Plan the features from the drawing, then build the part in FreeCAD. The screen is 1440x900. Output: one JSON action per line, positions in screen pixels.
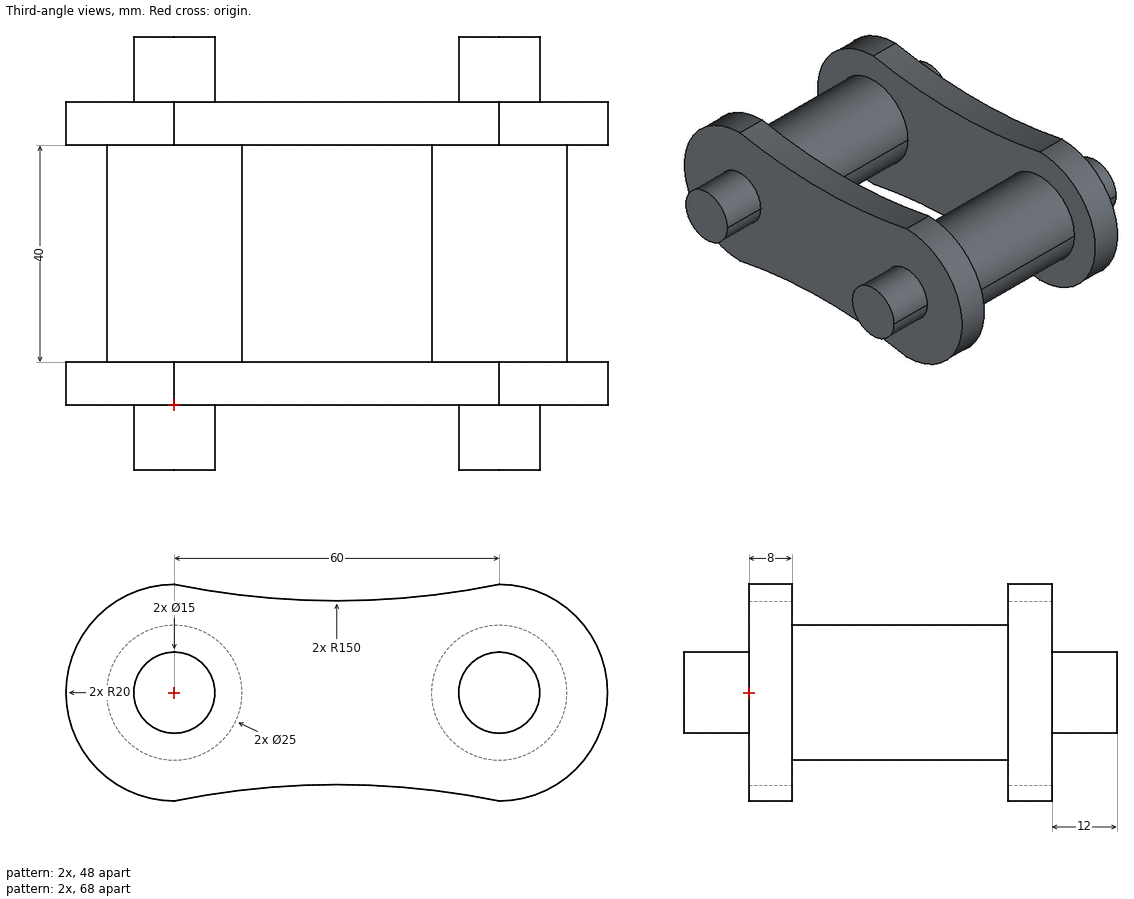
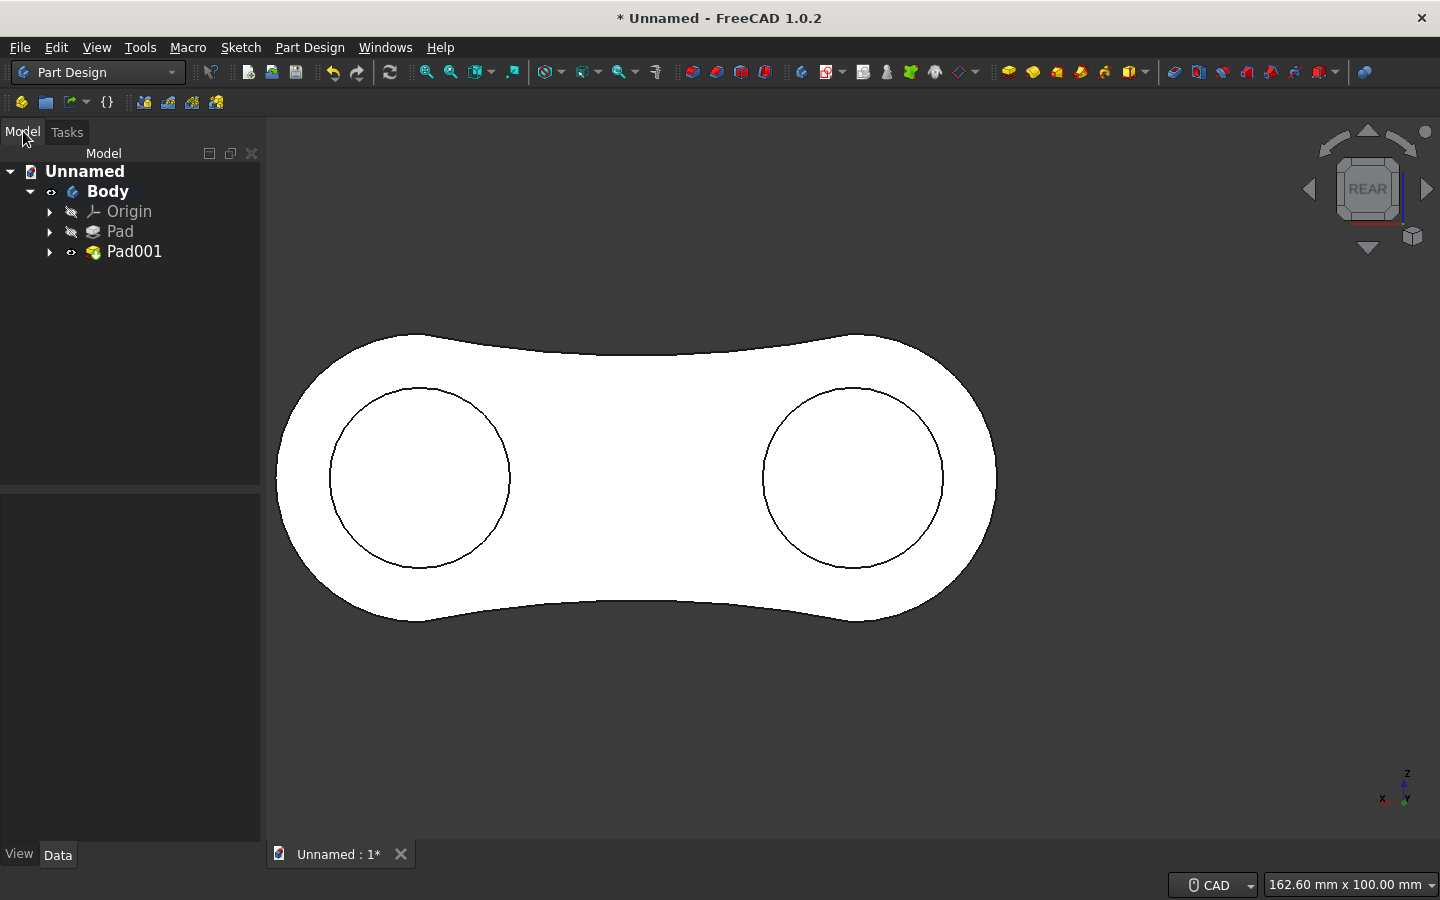
{"action": "left_click", "coordinate": [116, 232]}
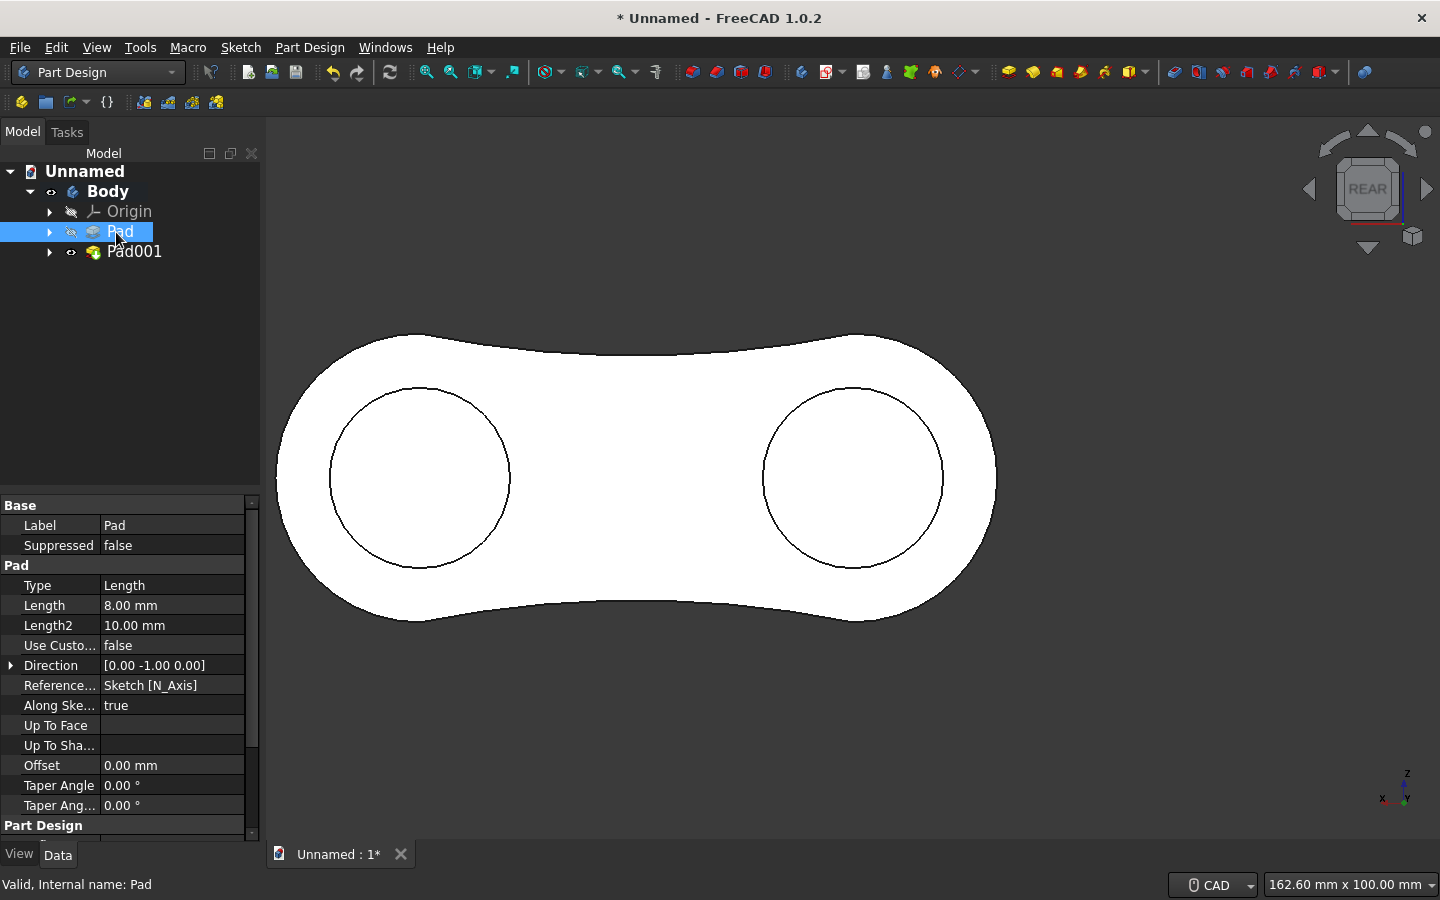
{"action": "left_click", "coordinate": [168, 102]}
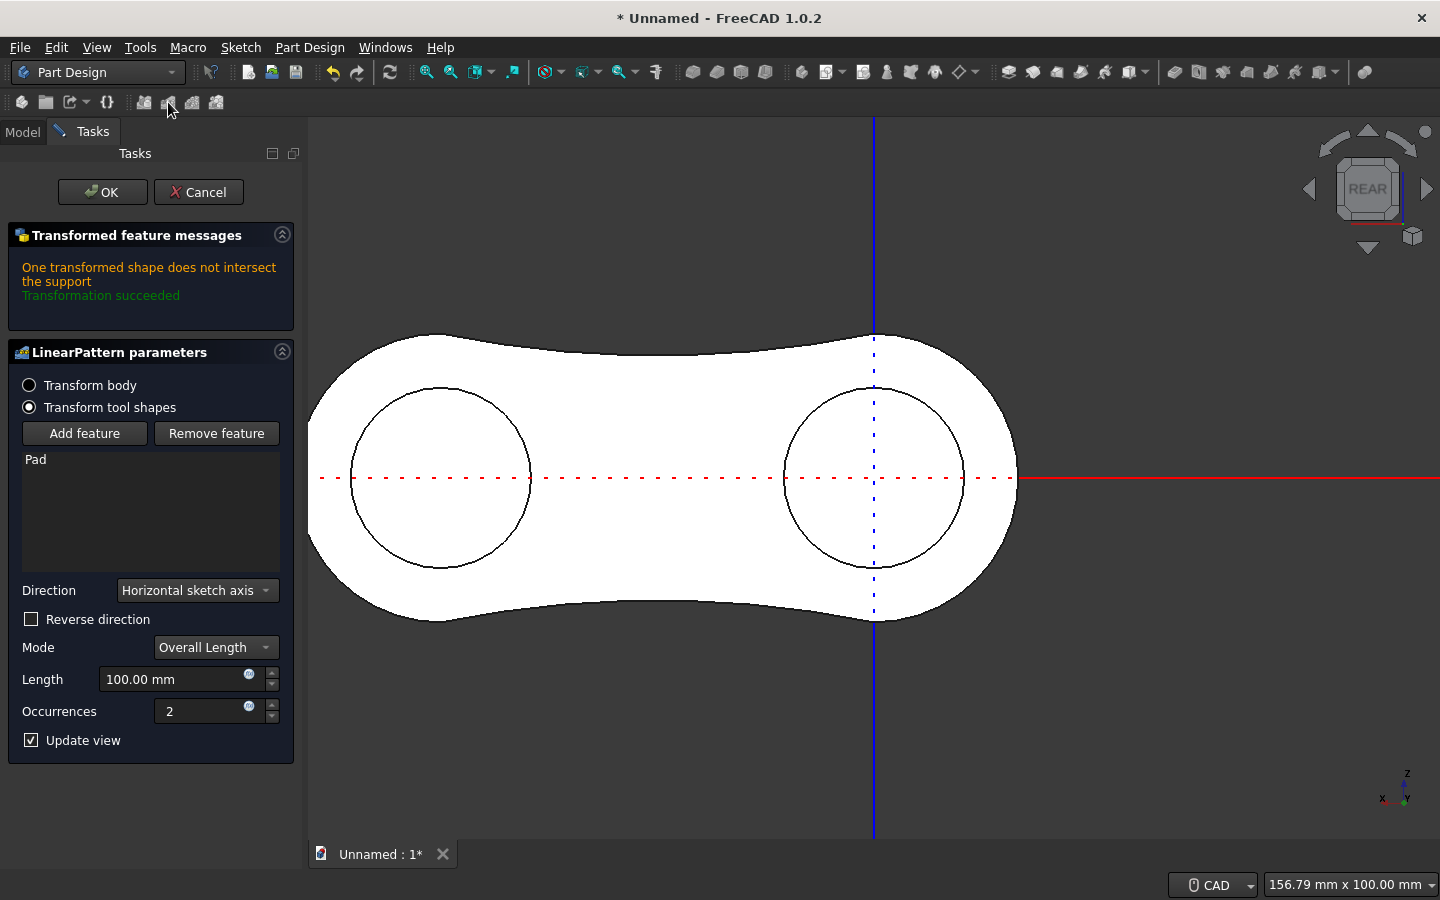
{"action": "left_click", "coordinate": [198, 590]}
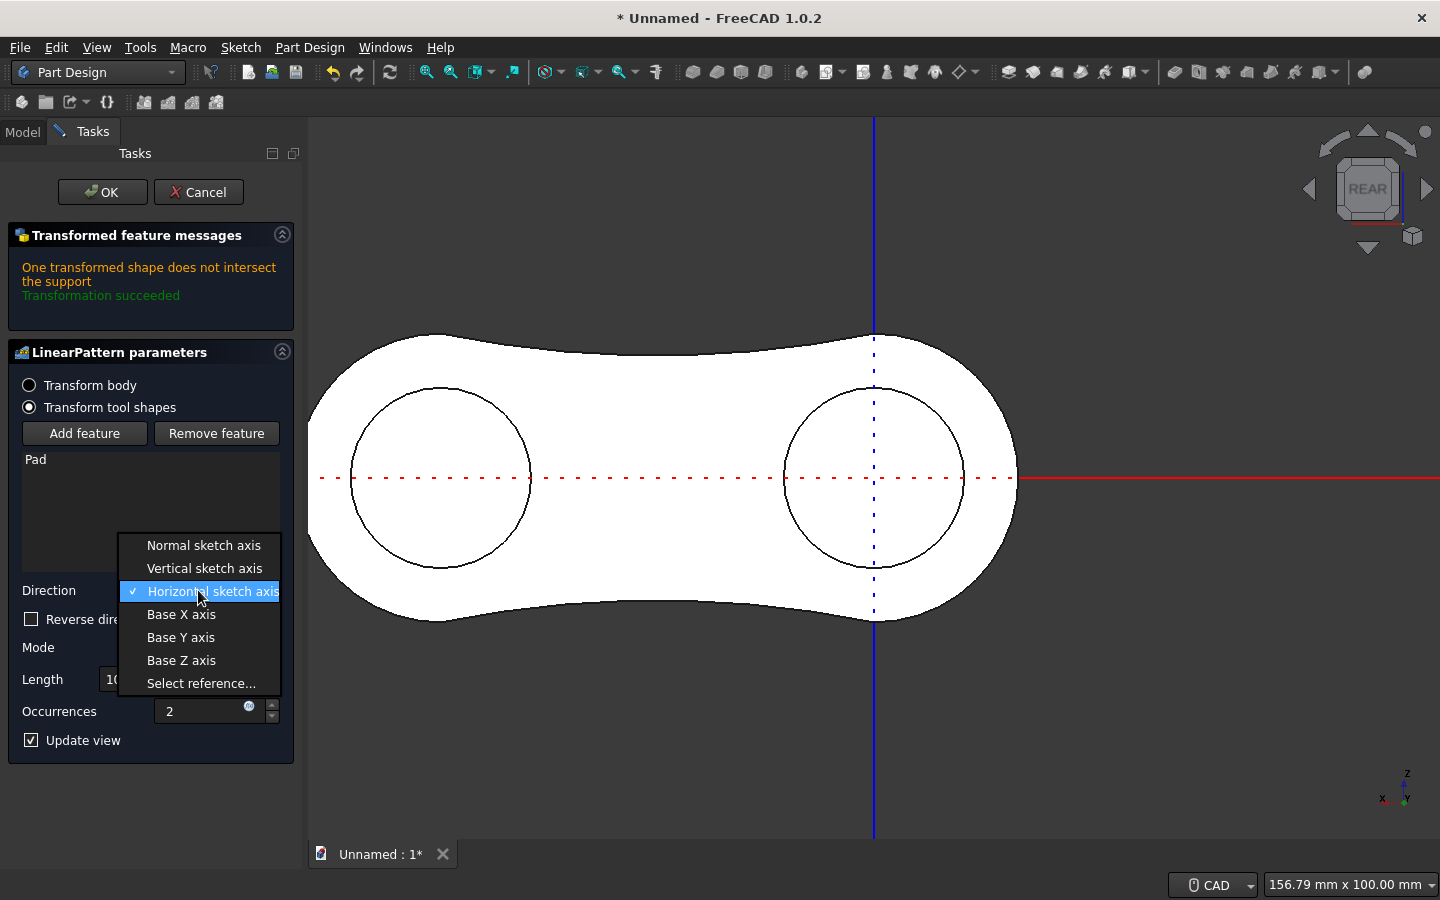
{"action": "left_click", "coordinate": [198, 638]}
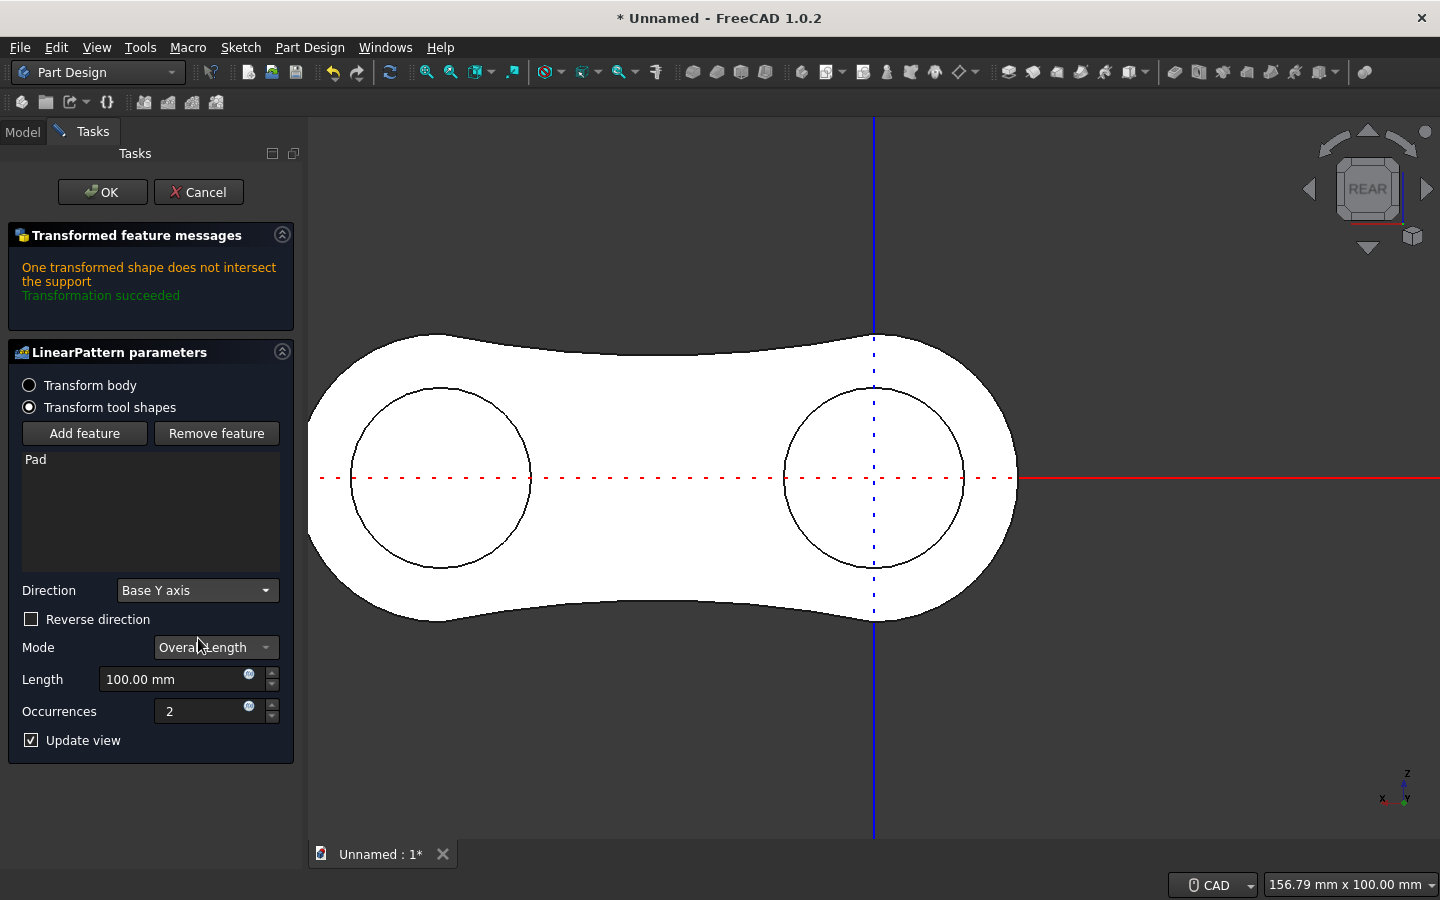
{"action": "left_click", "coordinate": [217, 648]}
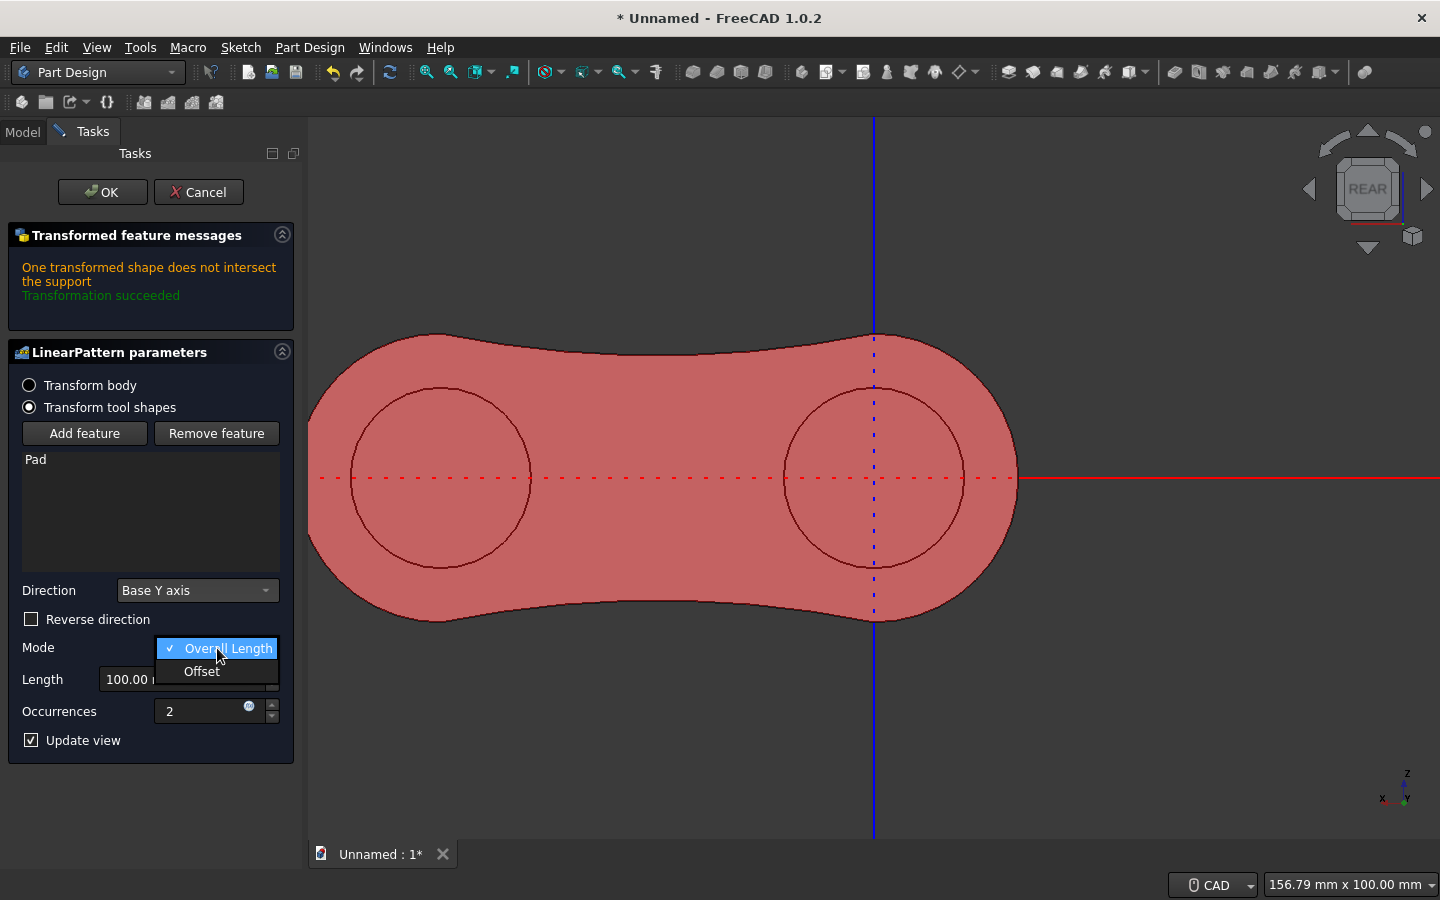
{"action": "left_click", "coordinate": [216, 672]}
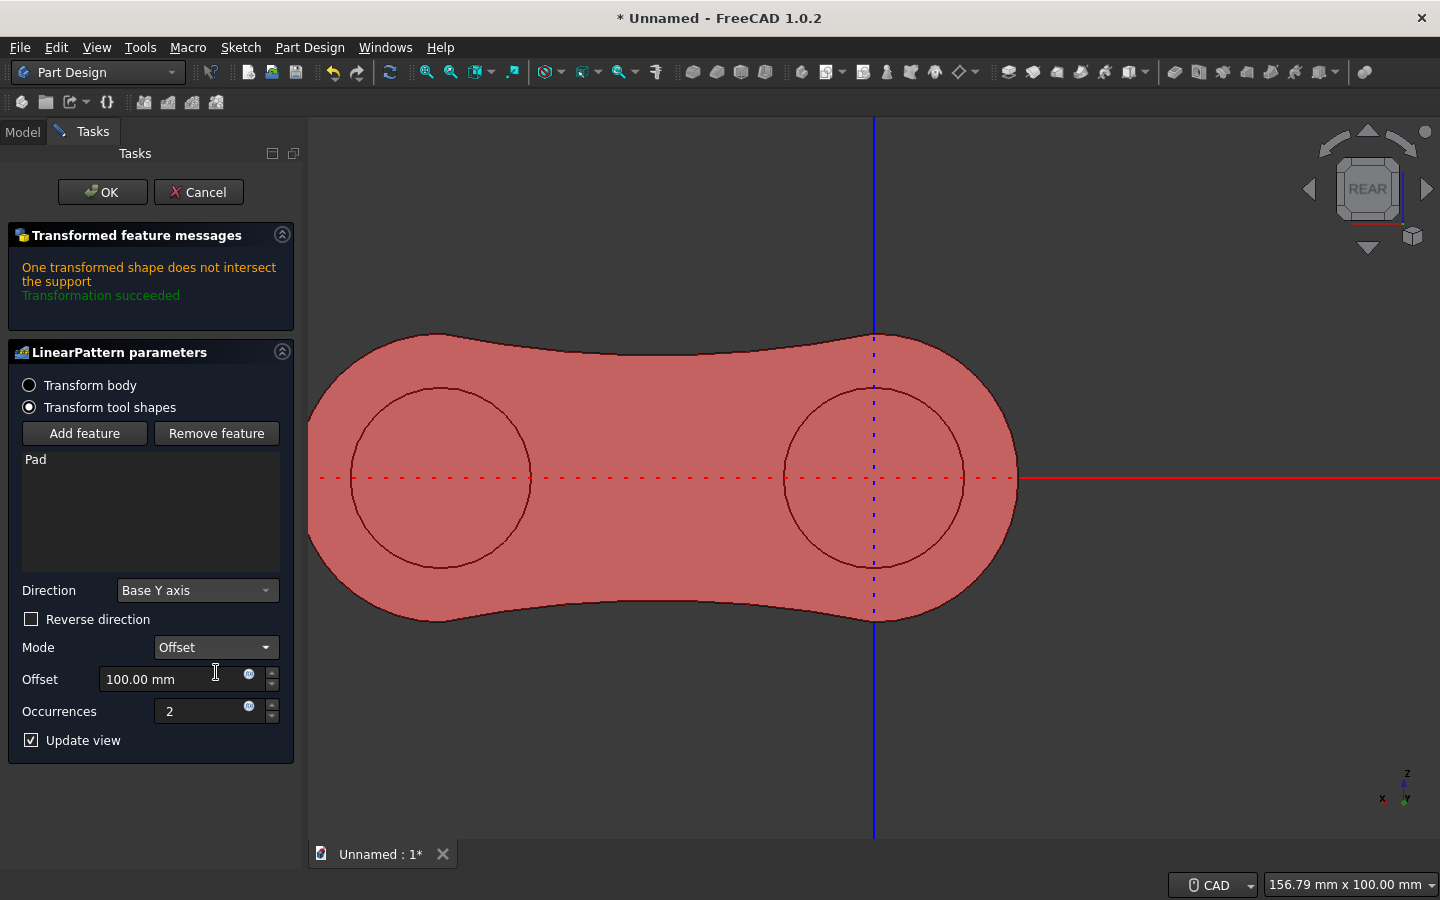
{"action": "triple_click", "coordinate": [182, 679]}